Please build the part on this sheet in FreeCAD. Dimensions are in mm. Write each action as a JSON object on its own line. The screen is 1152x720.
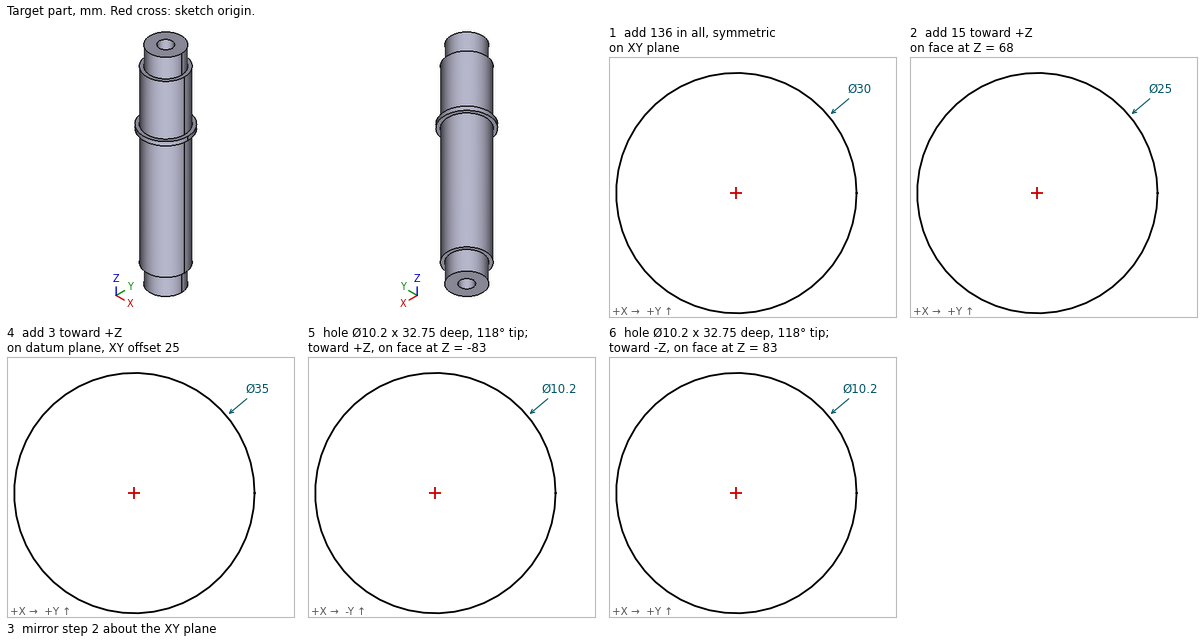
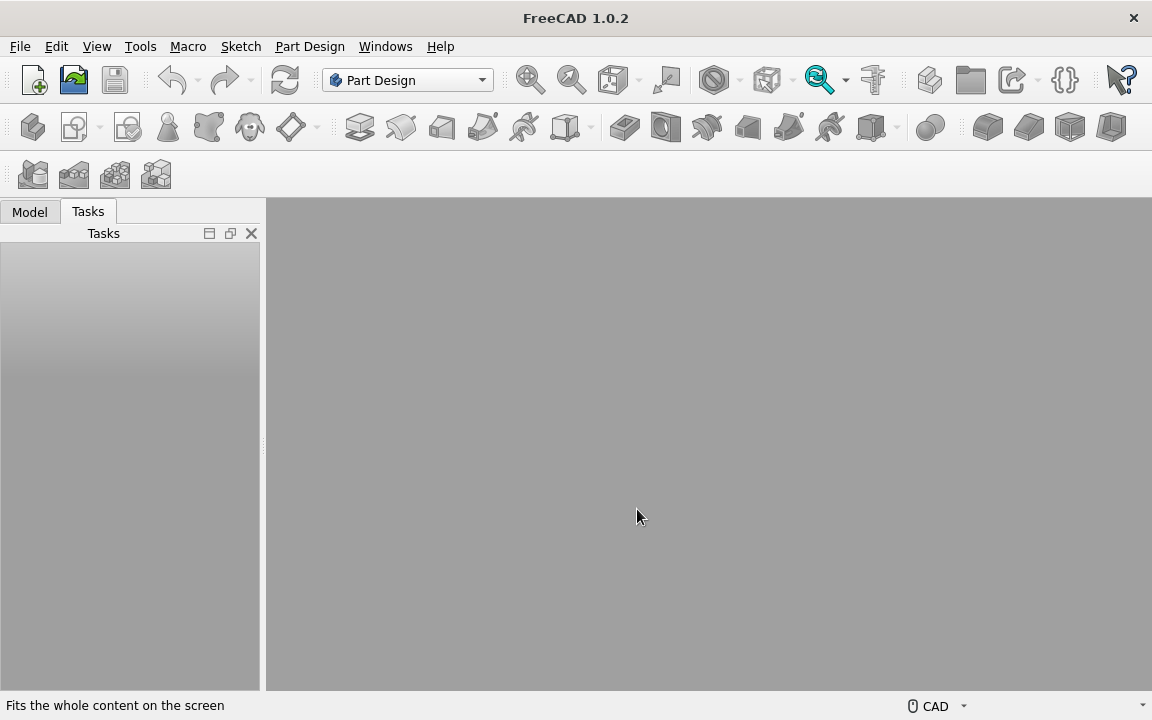
{"action": "left_click", "coordinate": [33, 80]}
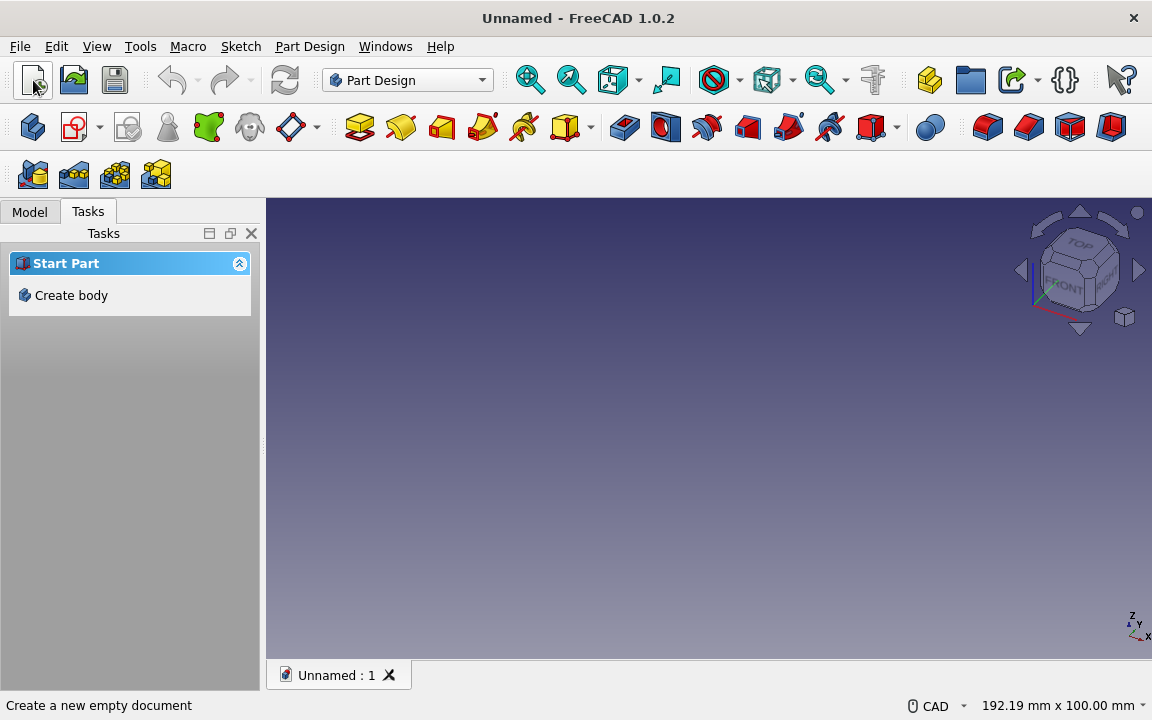
{"action": "left_click", "coordinate": [74, 128]}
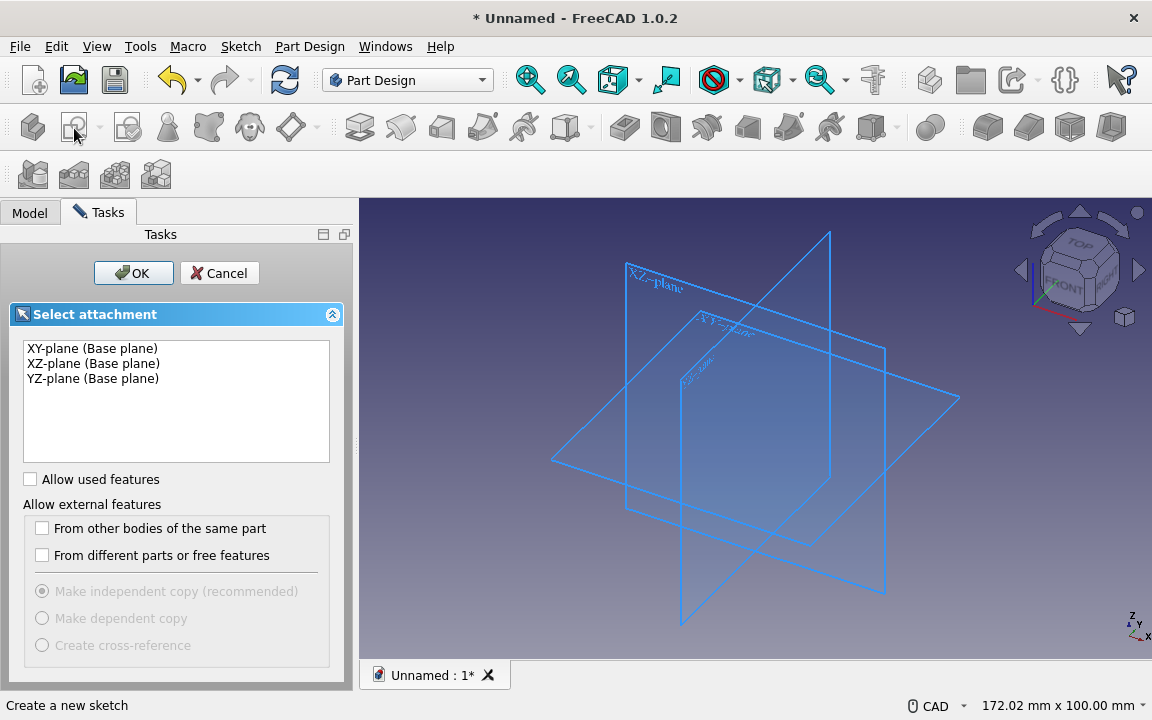
{"action": "left_click", "coordinate": [84, 348]}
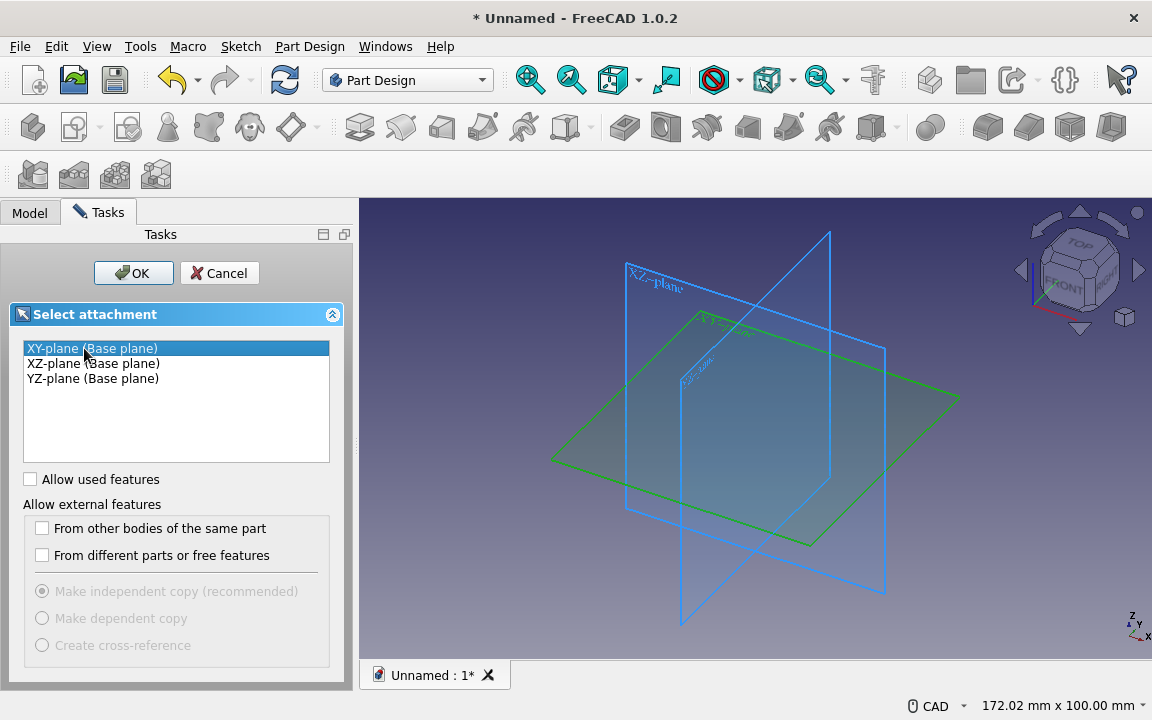
{"action": "left_click", "coordinate": [134, 273]}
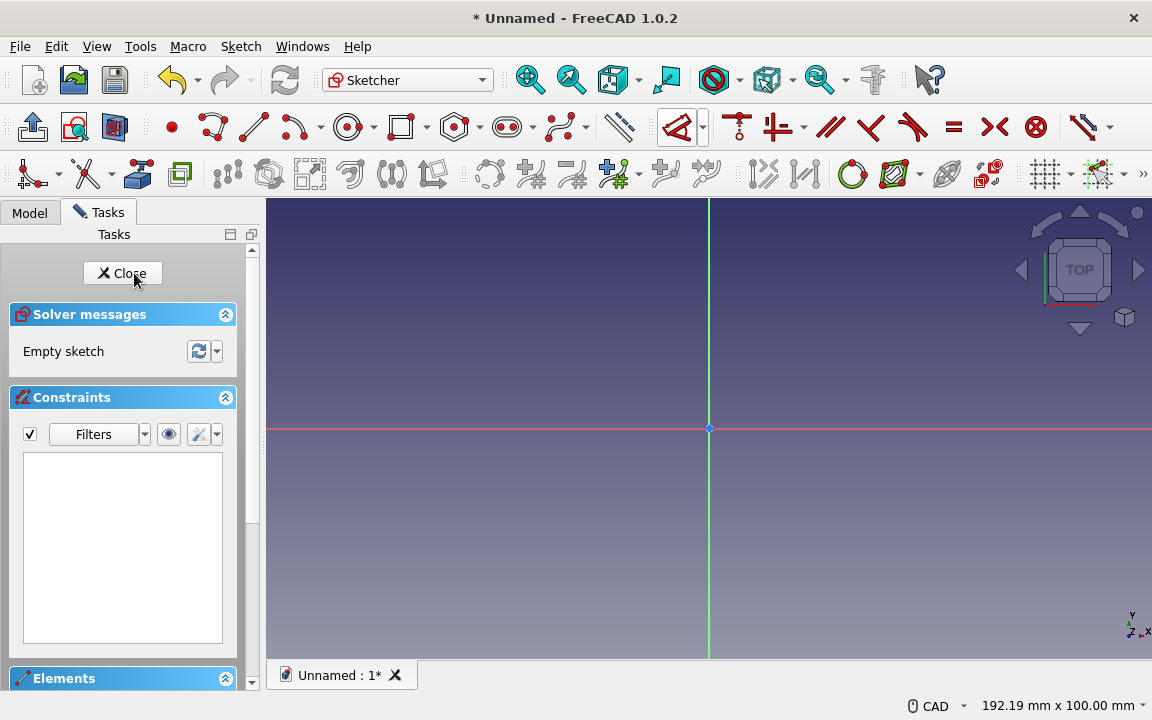
{"action": "scroll", "coordinate": [765, 428], "scroll_direction": "up", "scroll_amount": 4}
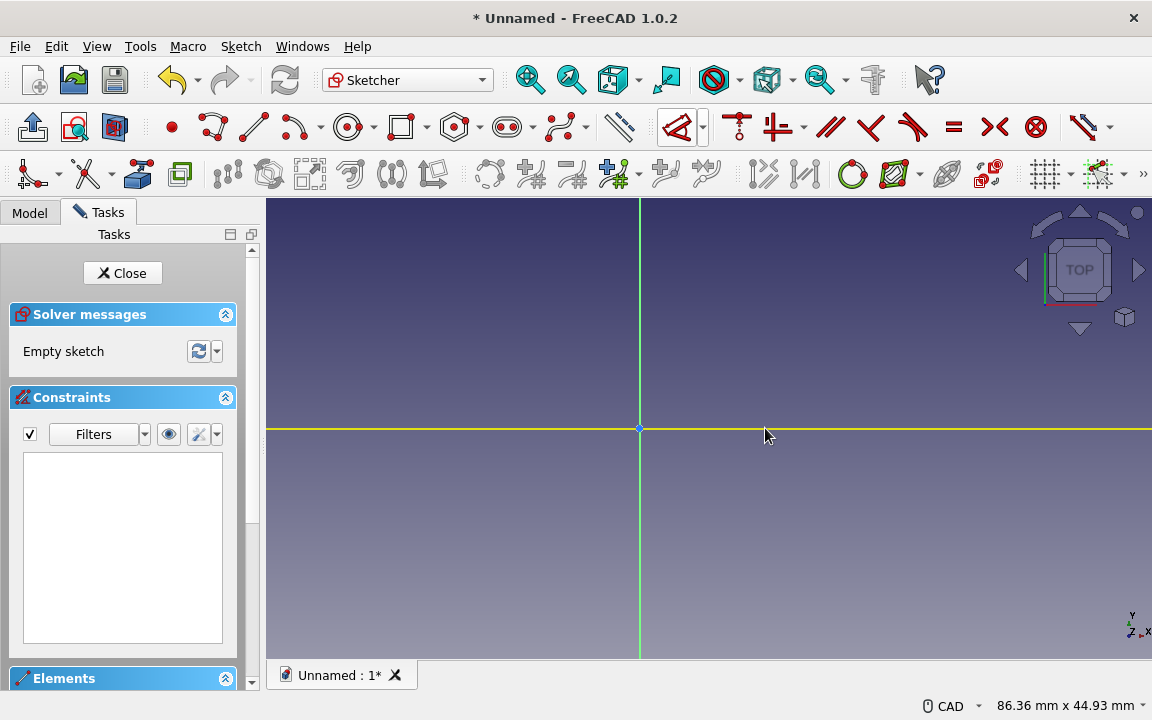
{"action": "left_click", "coordinate": [348, 128]}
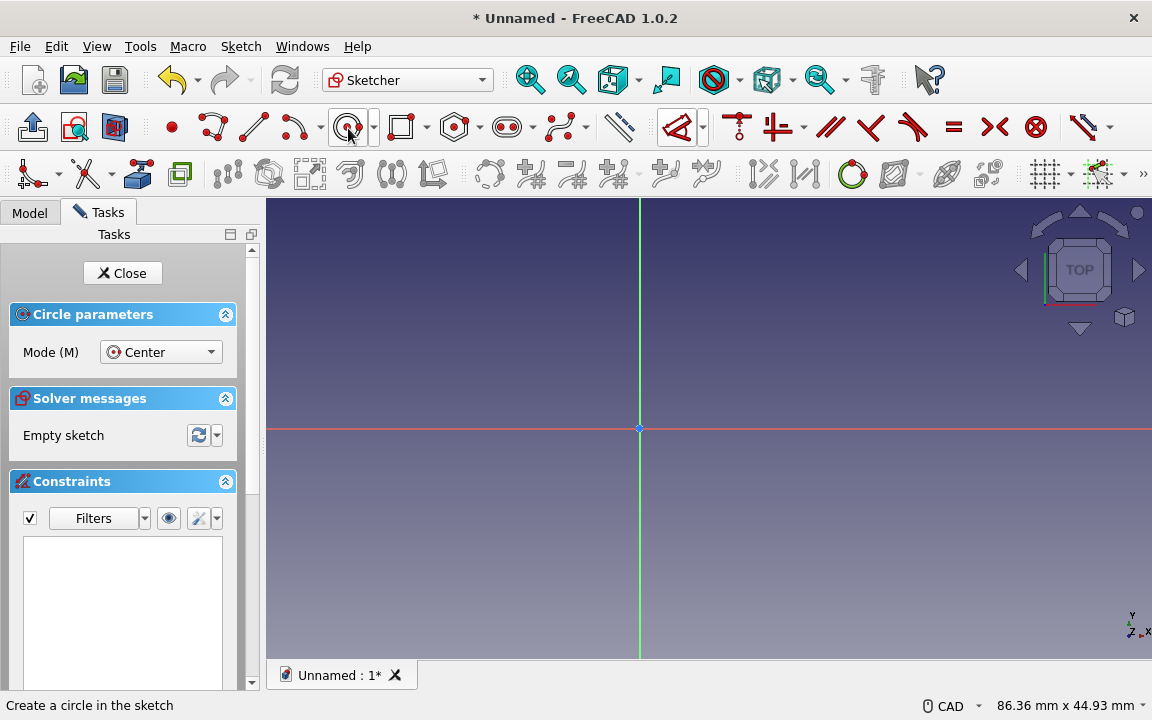
{"action": "left_click", "coordinate": [640, 428]}
{"action": "mouse_move", "coordinate": [748, 320]}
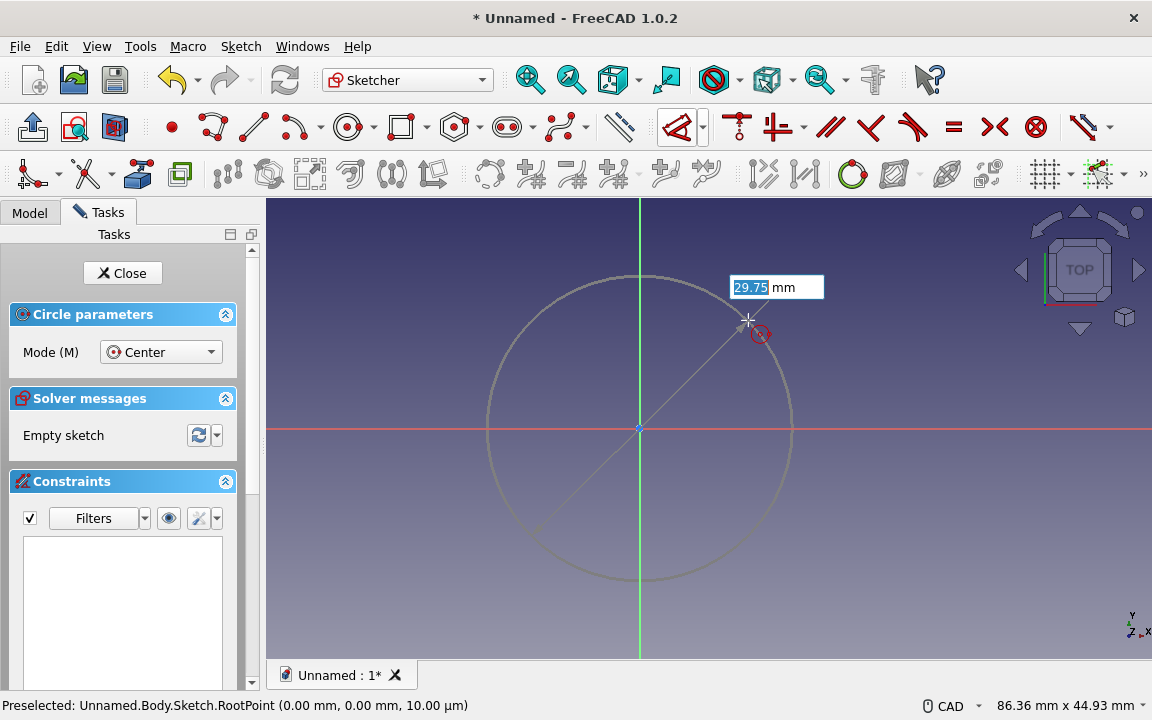
{"action": "type", "text": "30"}
{"action": "key", "text": "Return"}
{"action": "key", "text": "Escape"}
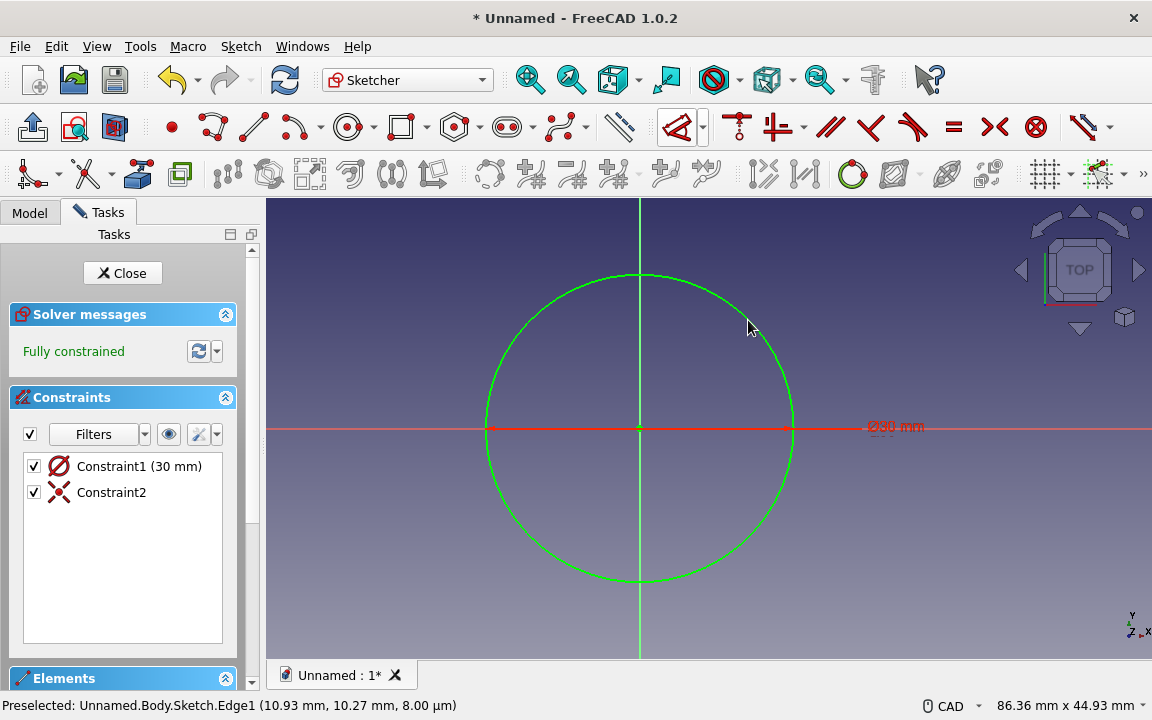
{"action": "left_click", "coordinate": [123, 273]}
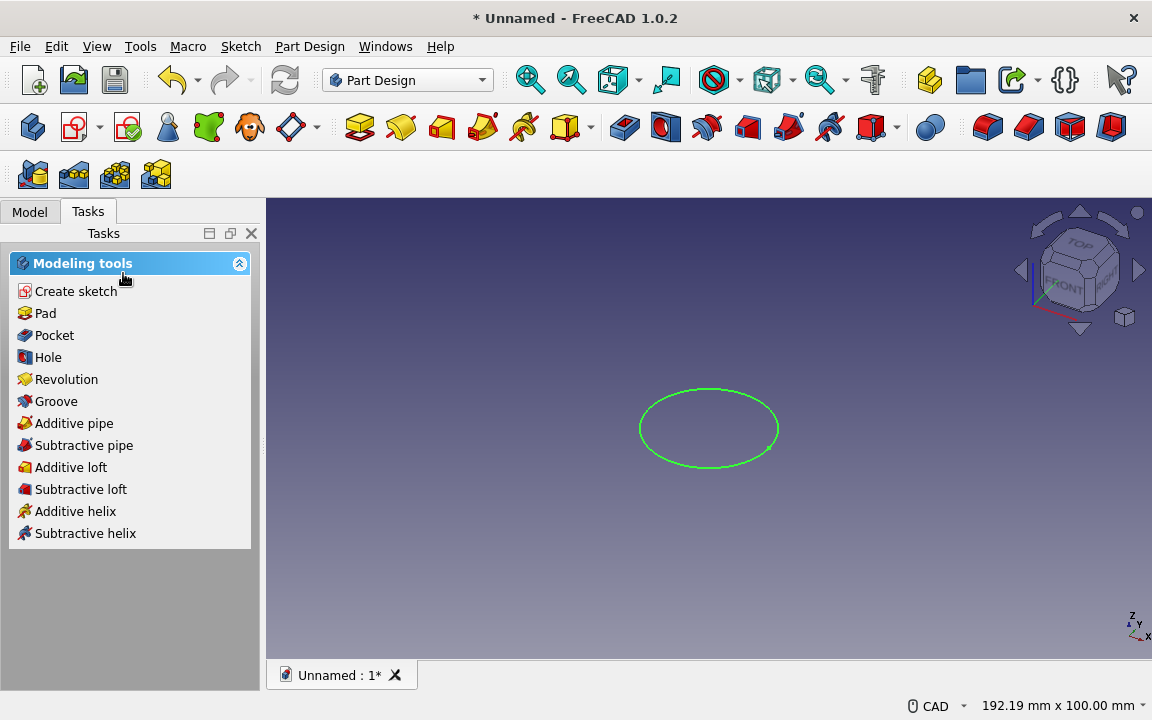
{"action": "left_click", "coordinate": [360, 128]}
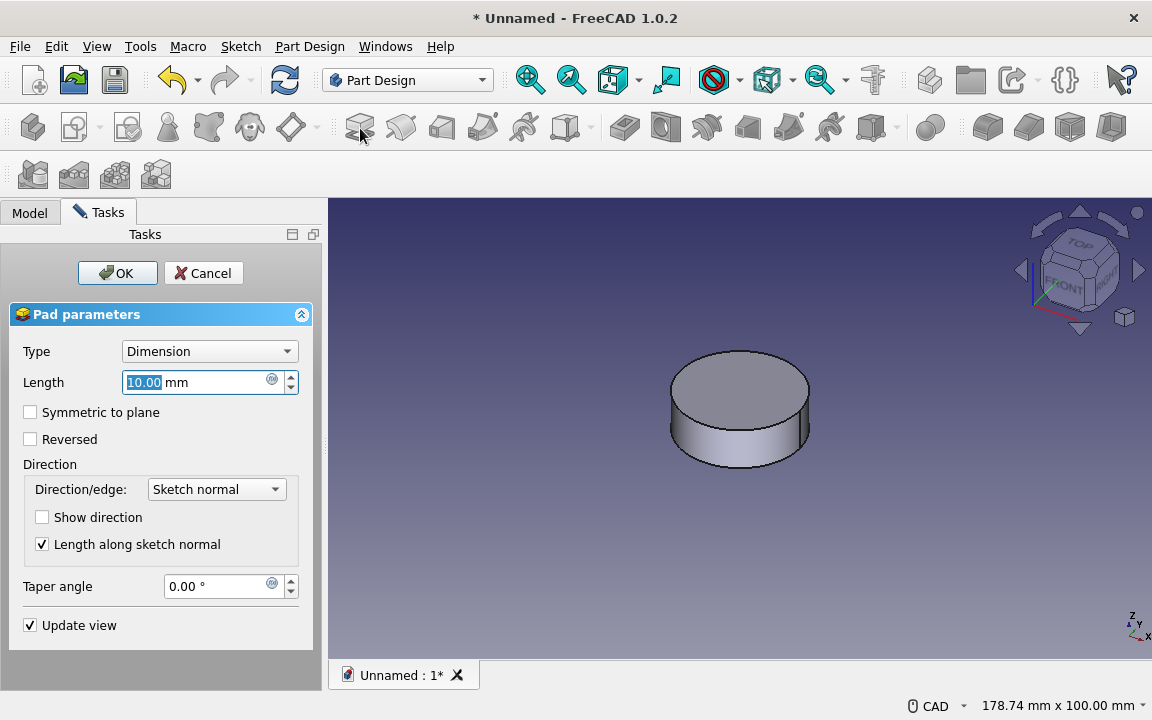
{"action": "type", "text": "136"}
{"action": "key", "text": "Tab"}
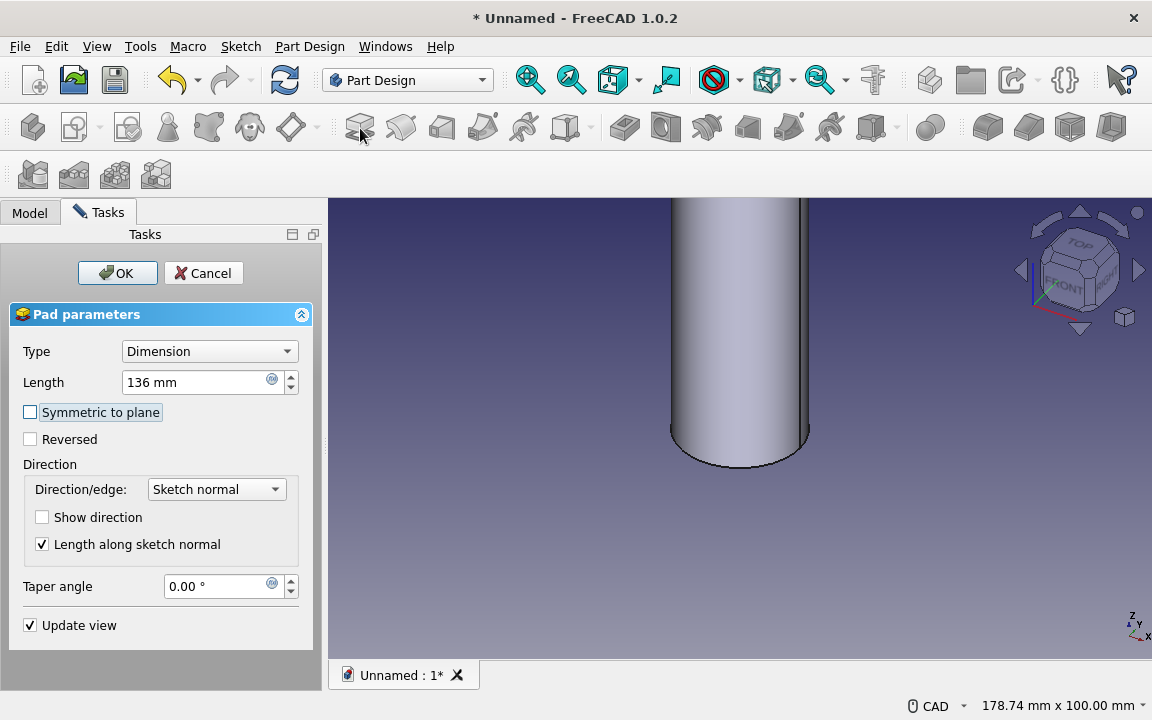
{"action": "left_click", "coordinate": [31, 412]}